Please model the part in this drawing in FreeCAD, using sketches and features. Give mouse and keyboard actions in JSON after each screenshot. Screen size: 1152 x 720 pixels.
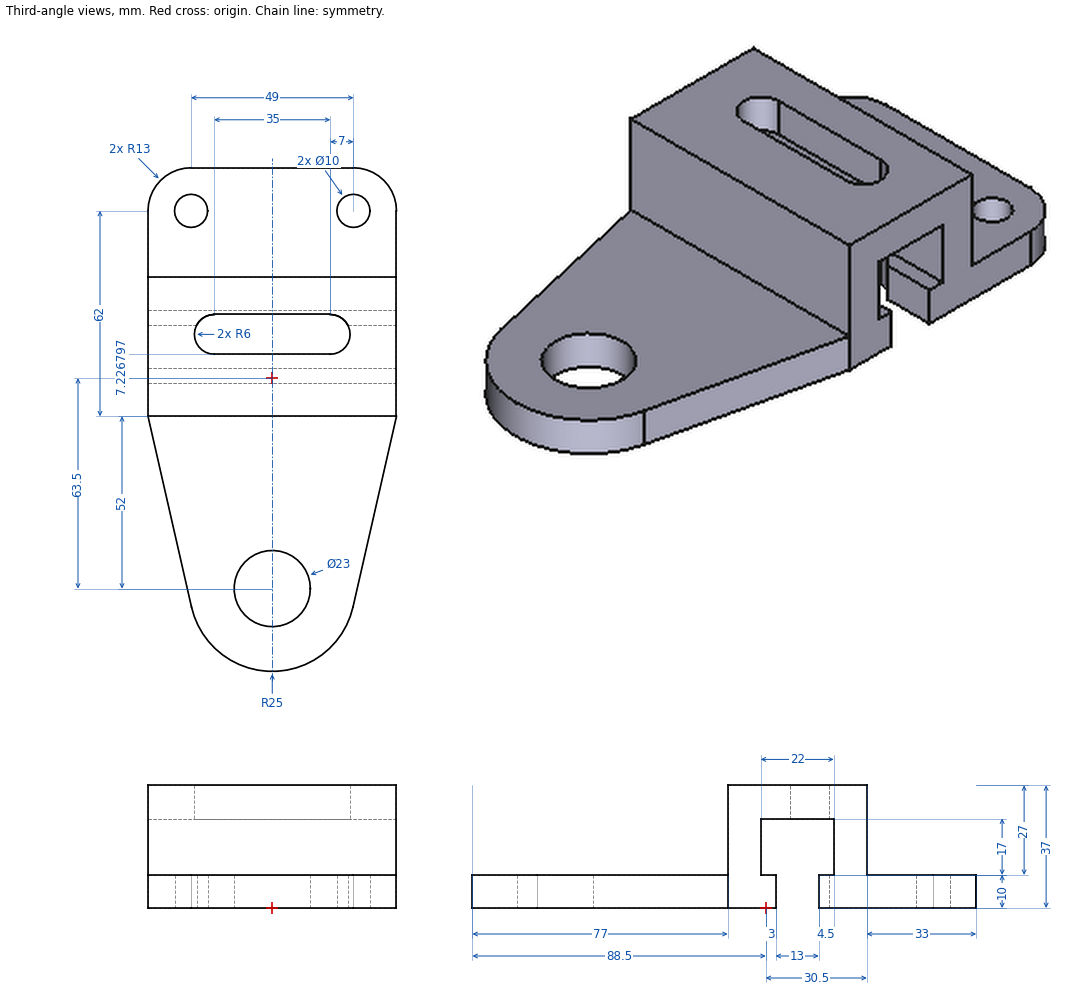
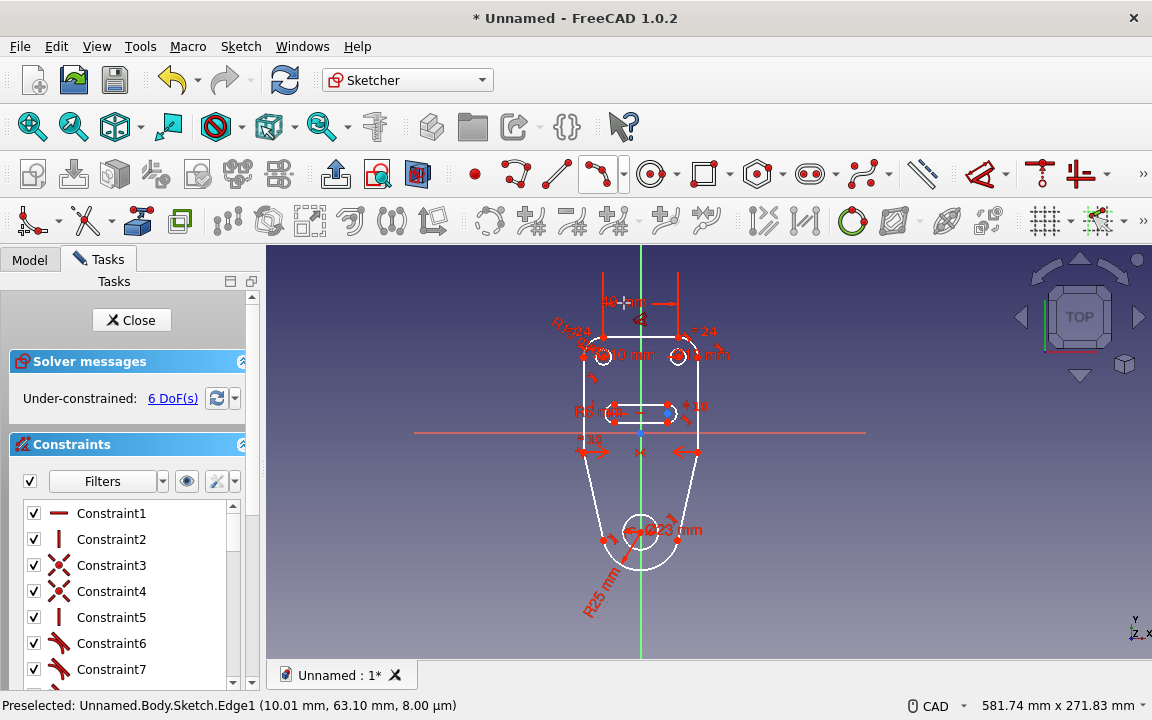
{"action": "left_click", "coordinate": [584, 386]}
{"action": "left_click", "coordinate": [550, 383]}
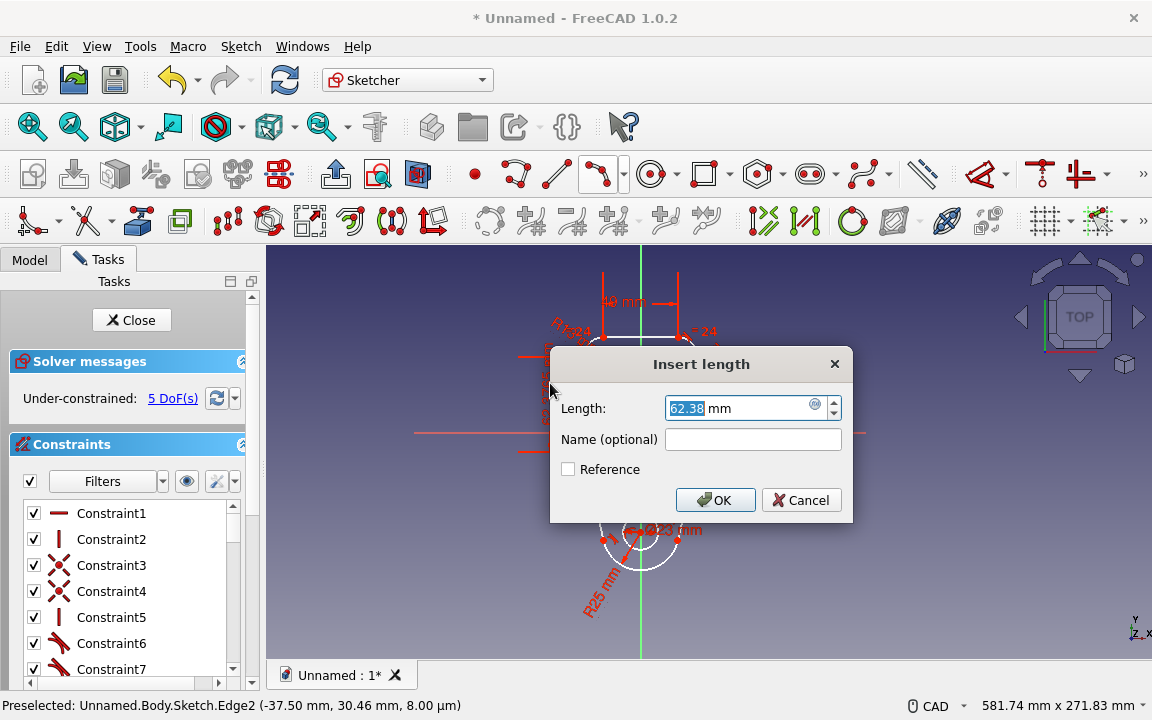
{"action": "type", "text": "62"}
{"action": "key", "text": "Return"}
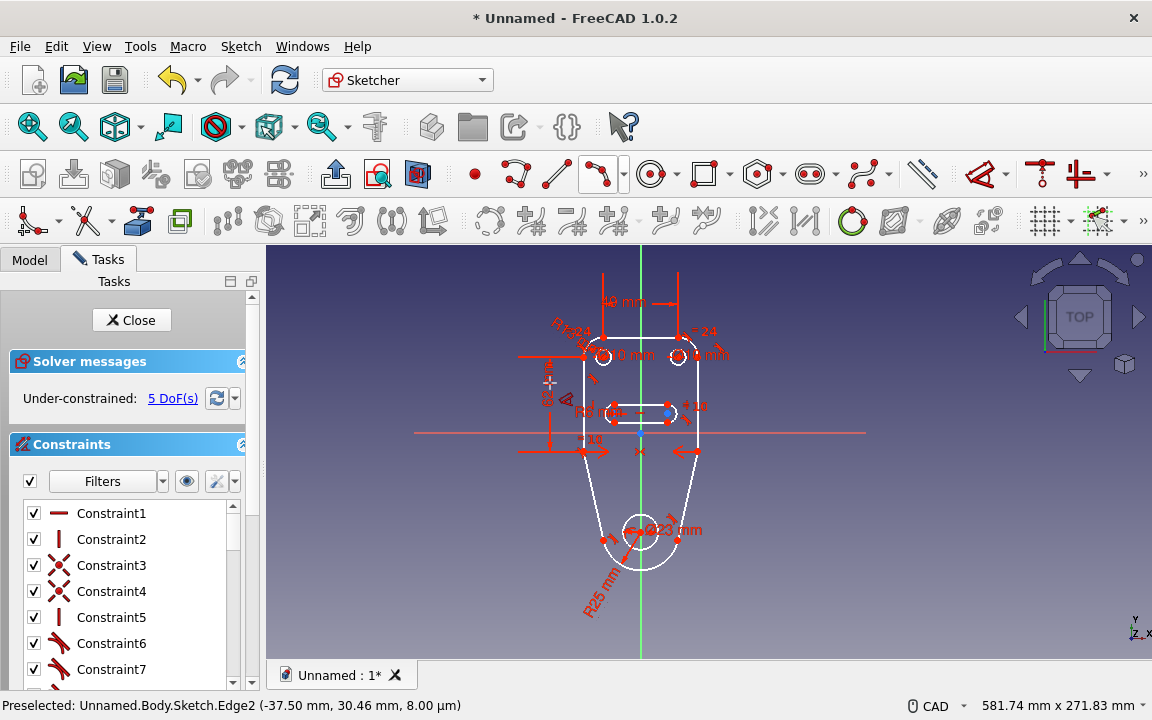
{"action": "scroll", "coordinate": [630, 405], "scroll_direction": "up", "scroll_amount": 2}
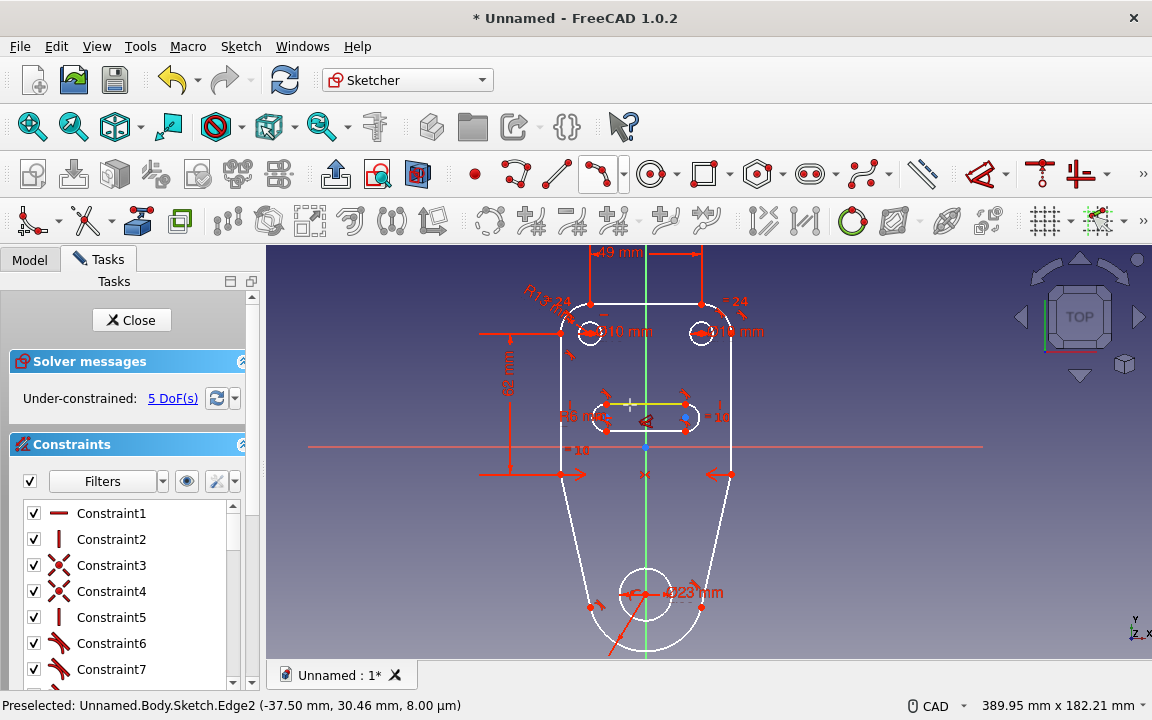
{"action": "left_click", "coordinate": [630, 404]}
{"action": "left_click", "coordinate": [628, 370]}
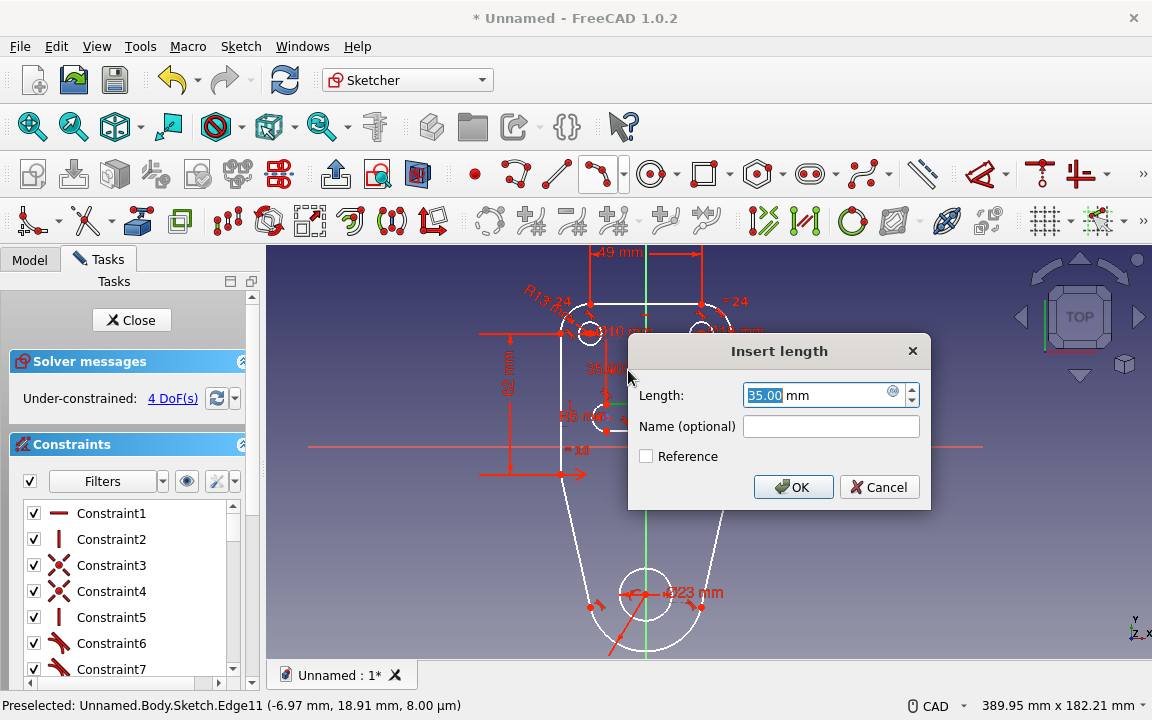
{"action": "type", "text": "35"}
{"action": "key", "text": "Return"}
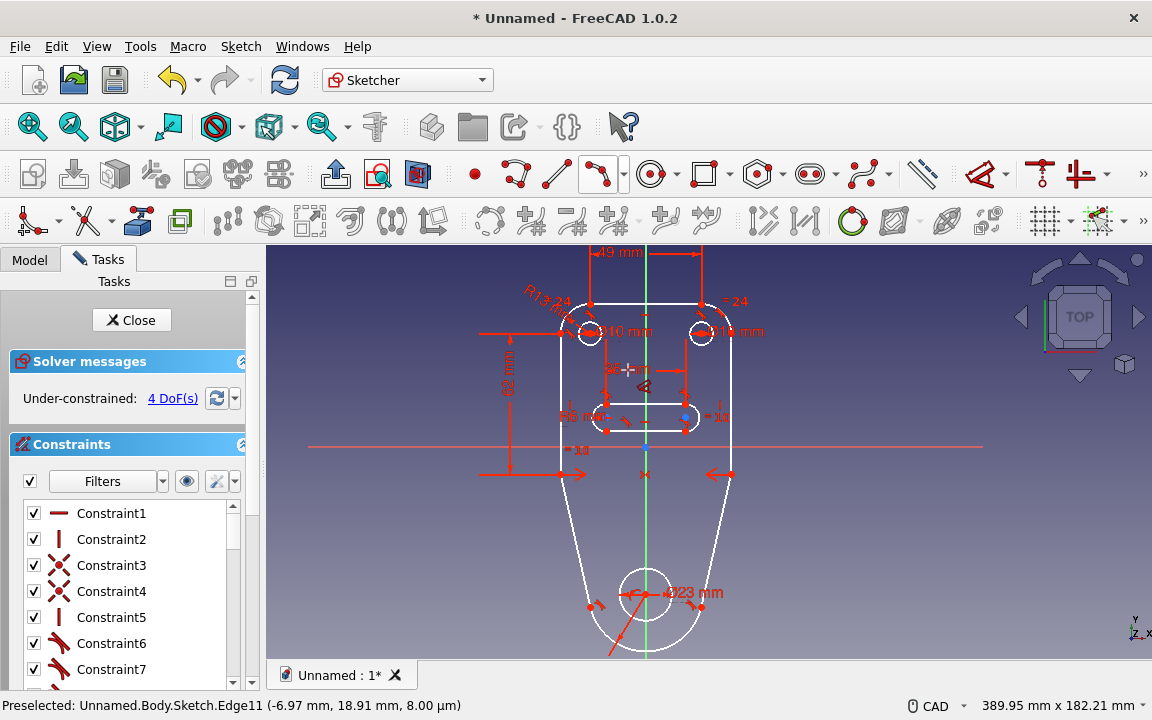
{"action": "scroll", "coordinate": [686, 404], "scroll_direction": "up", "scroll_amount": 5}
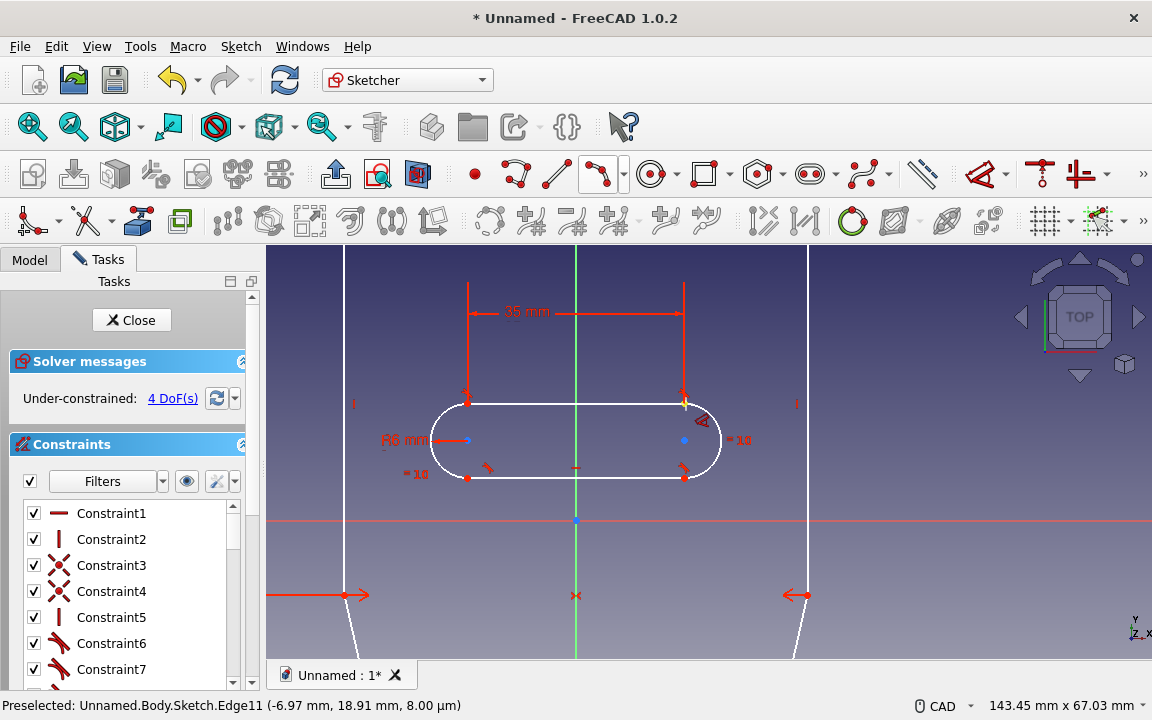
{"action": "left_click", "coordinate": [684, 404]}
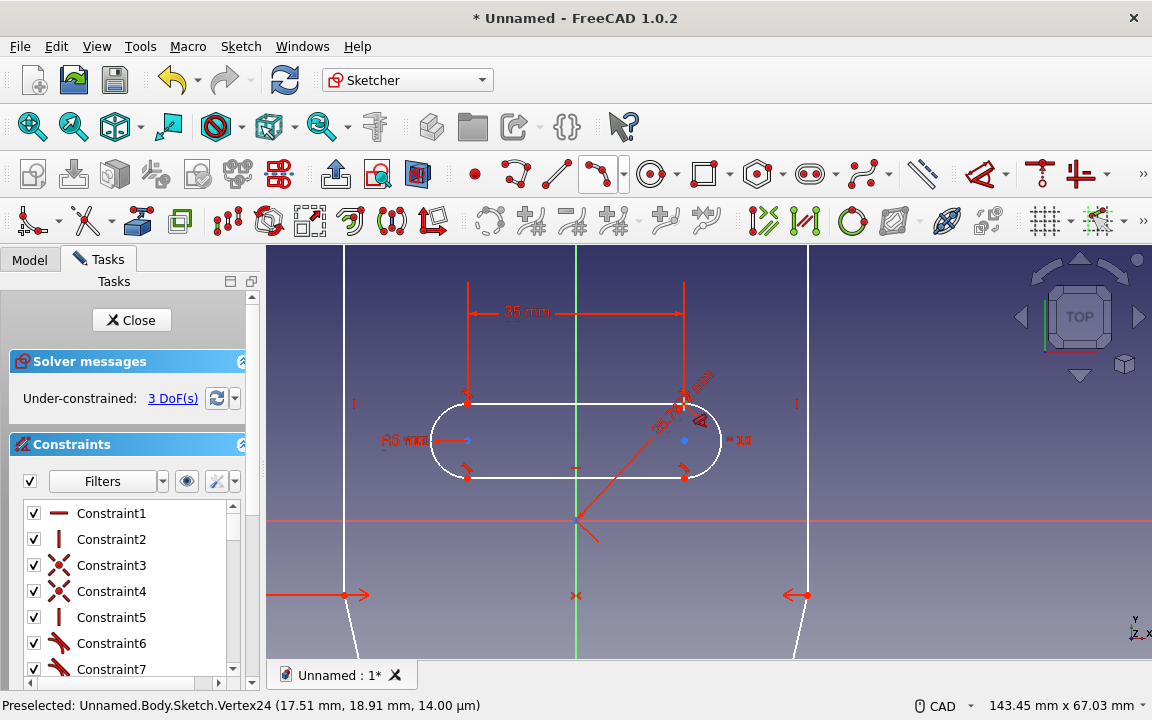
{"action": "scroll", "coordinate": [662, 404], "scroll_direction": "down", "scroll_amount": 7}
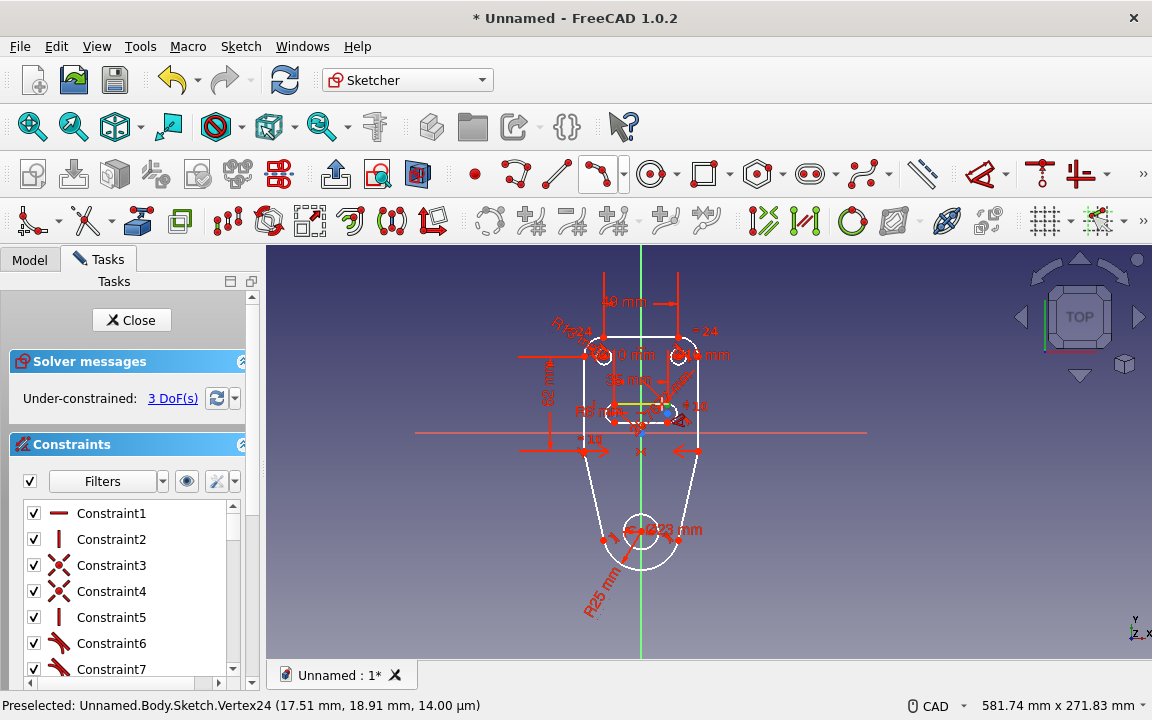
{"action": "scroll", "coordinate": [678, 357], "scroll_direction": "up", "scroll_amount": 7}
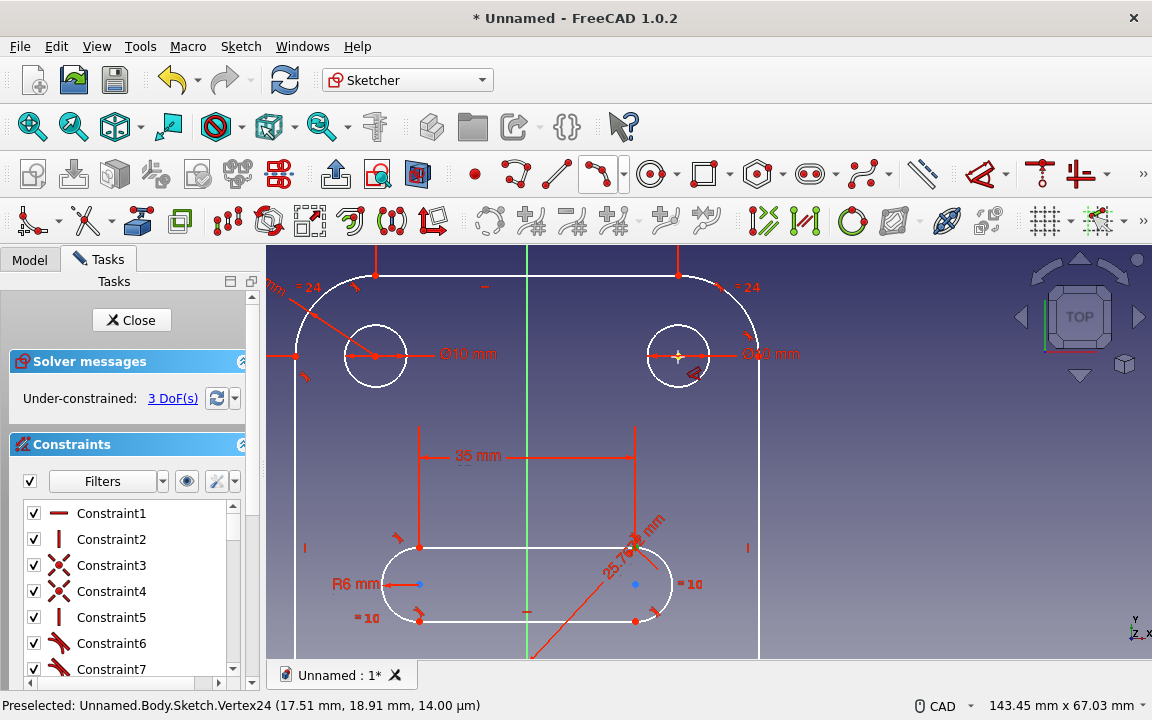
{"action": "left_click", "coordinate": [678, 356]}
{"action": "left_click", "coordinate": [647, 322]}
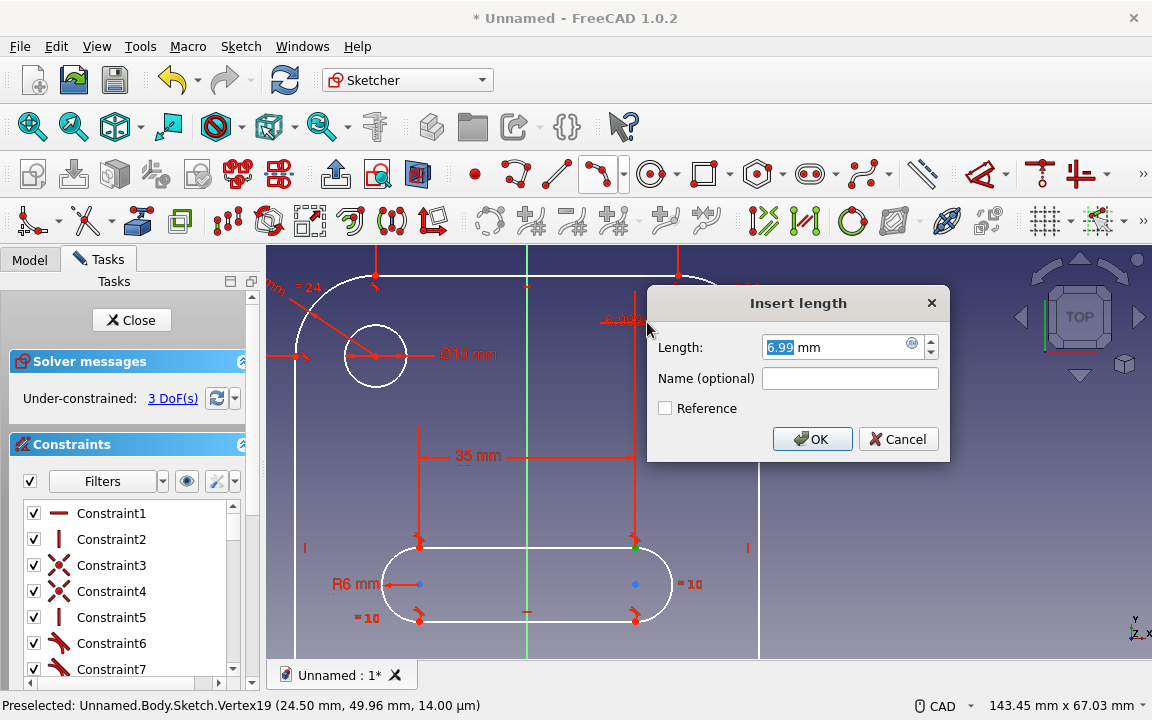
{"action": "type", "text": "7"}
{"action": "key", "text": "Return"}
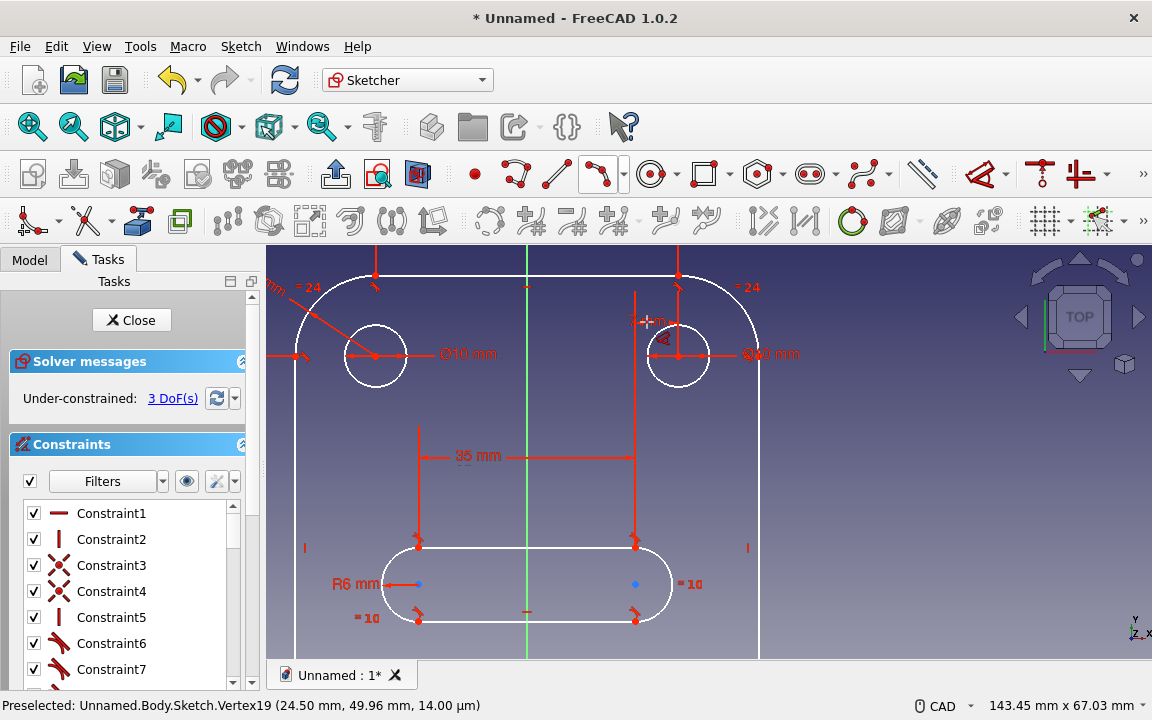
{"action": "scroll", "coordinate": [678, 357], "scroll_direction": "down", "scroll_amount": 7}